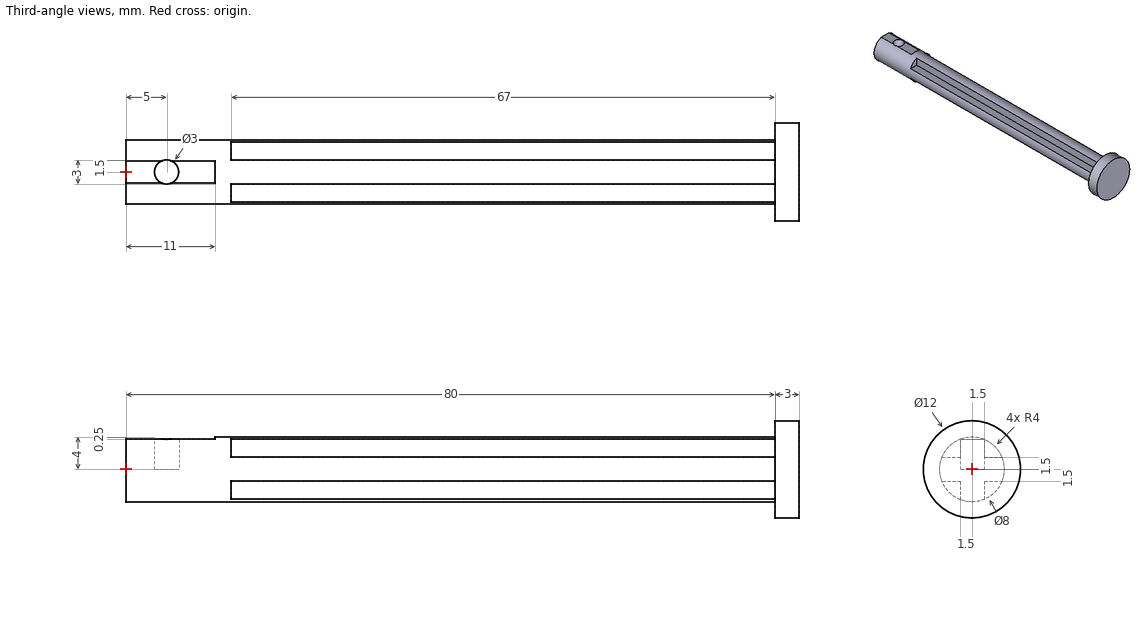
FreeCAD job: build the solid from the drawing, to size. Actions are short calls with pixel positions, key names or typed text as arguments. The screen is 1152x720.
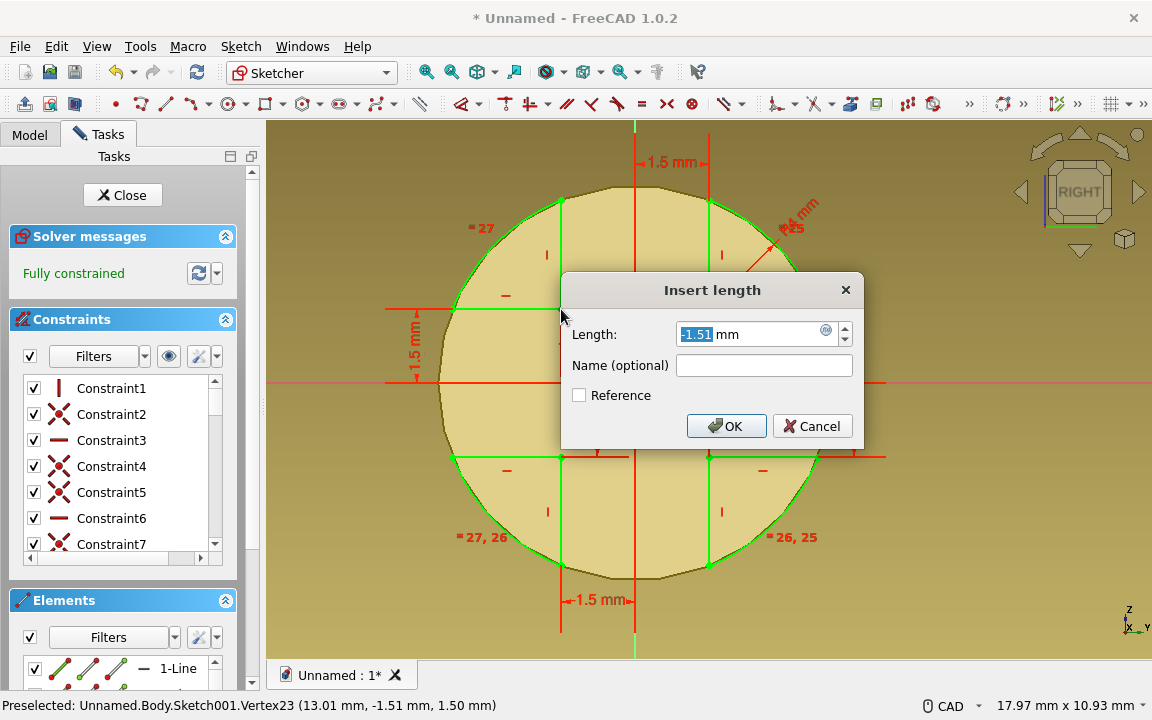
text(-1.5)
key(Return)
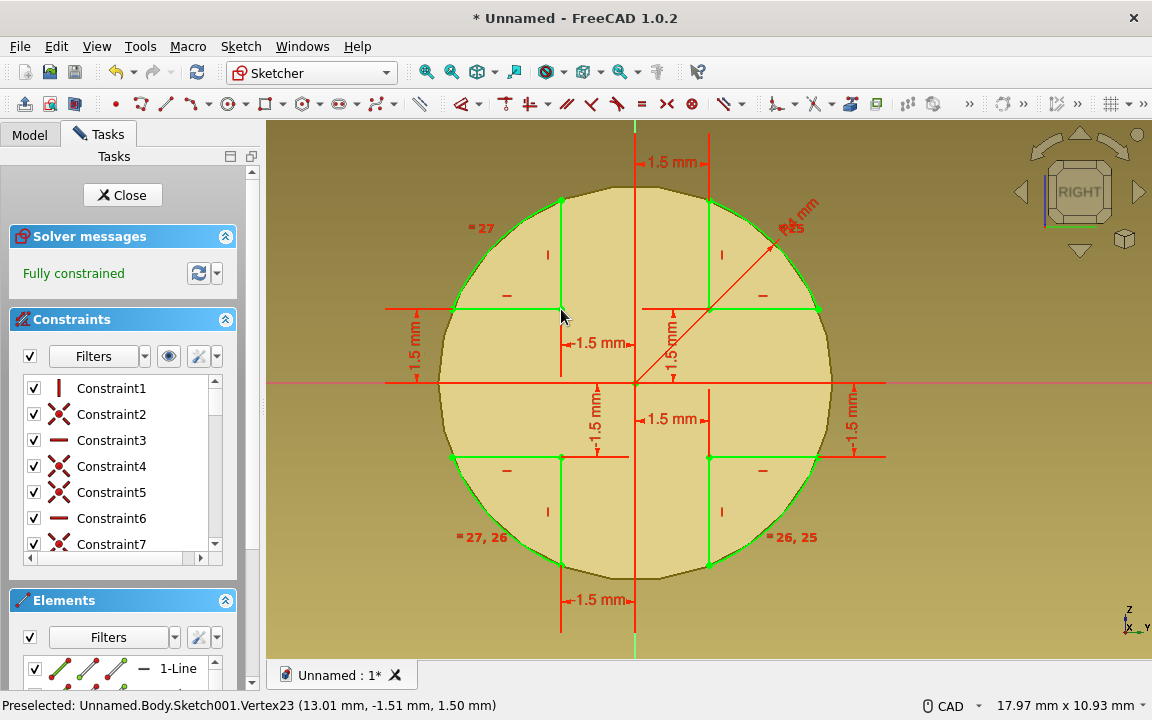
click(123, 195)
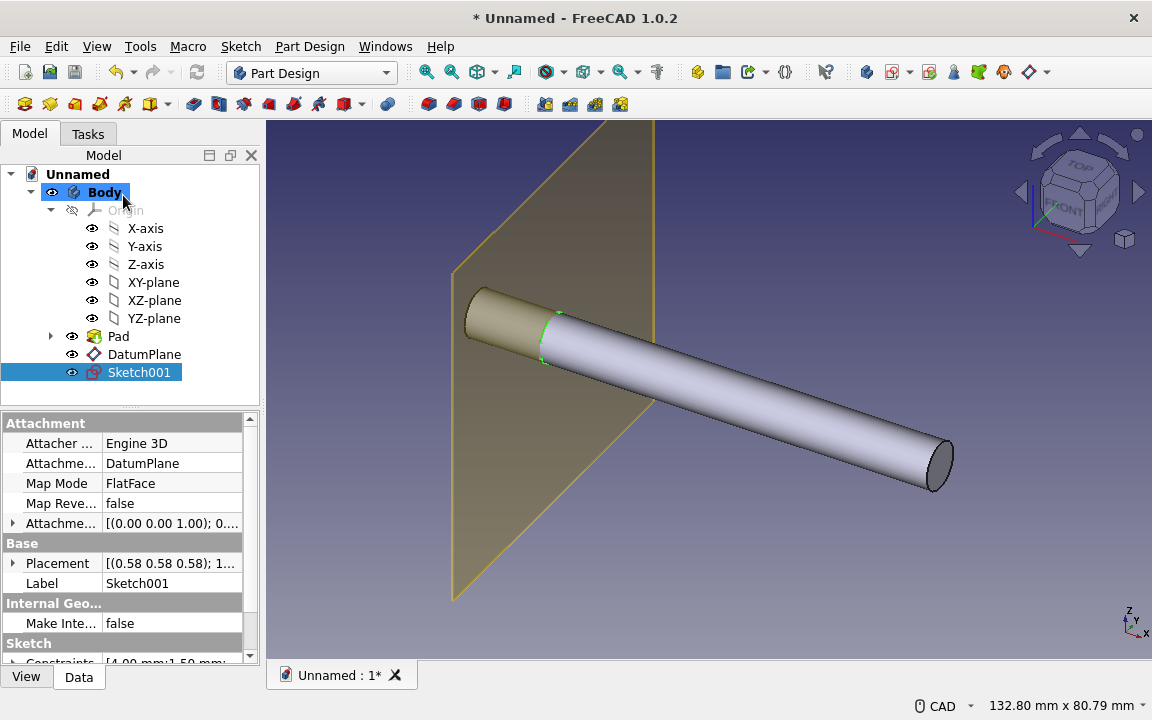
click(194, 104)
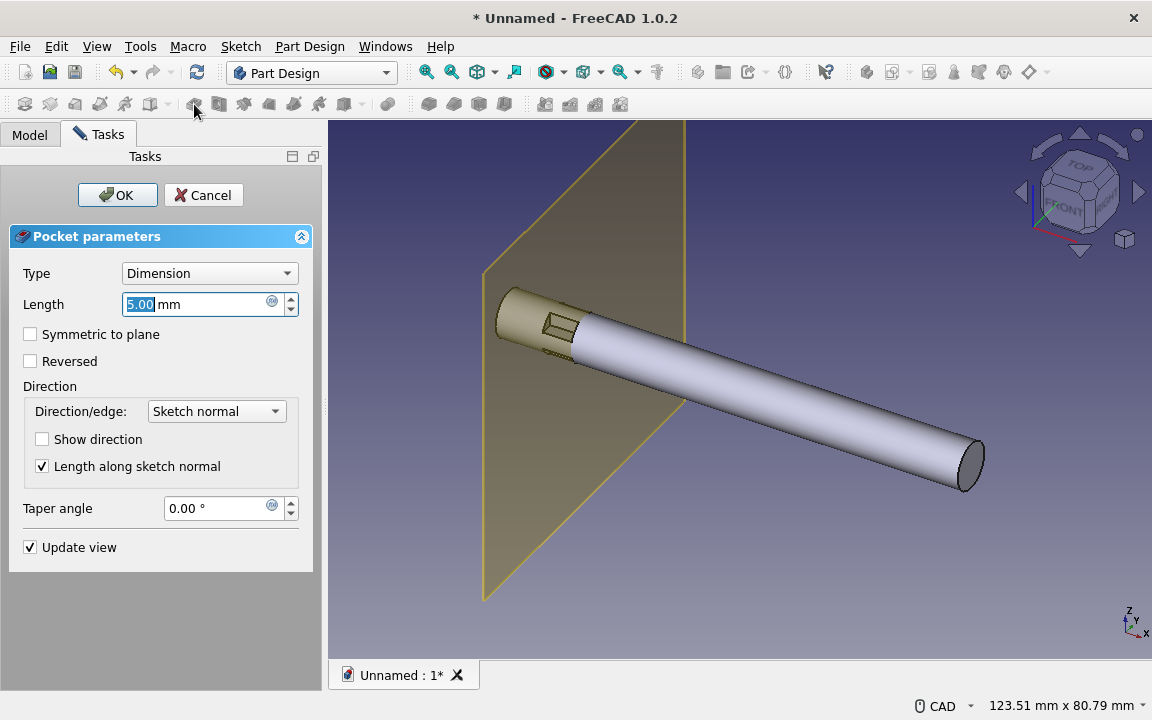
text(67)
key(Tab)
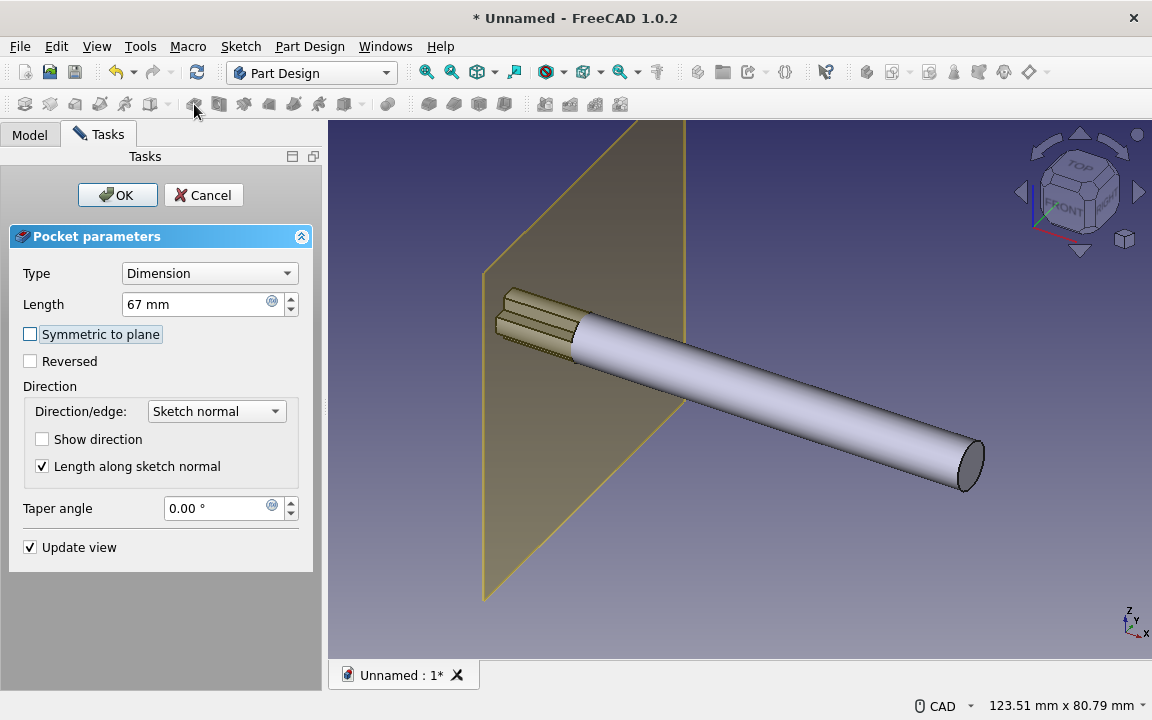
click(31, 361)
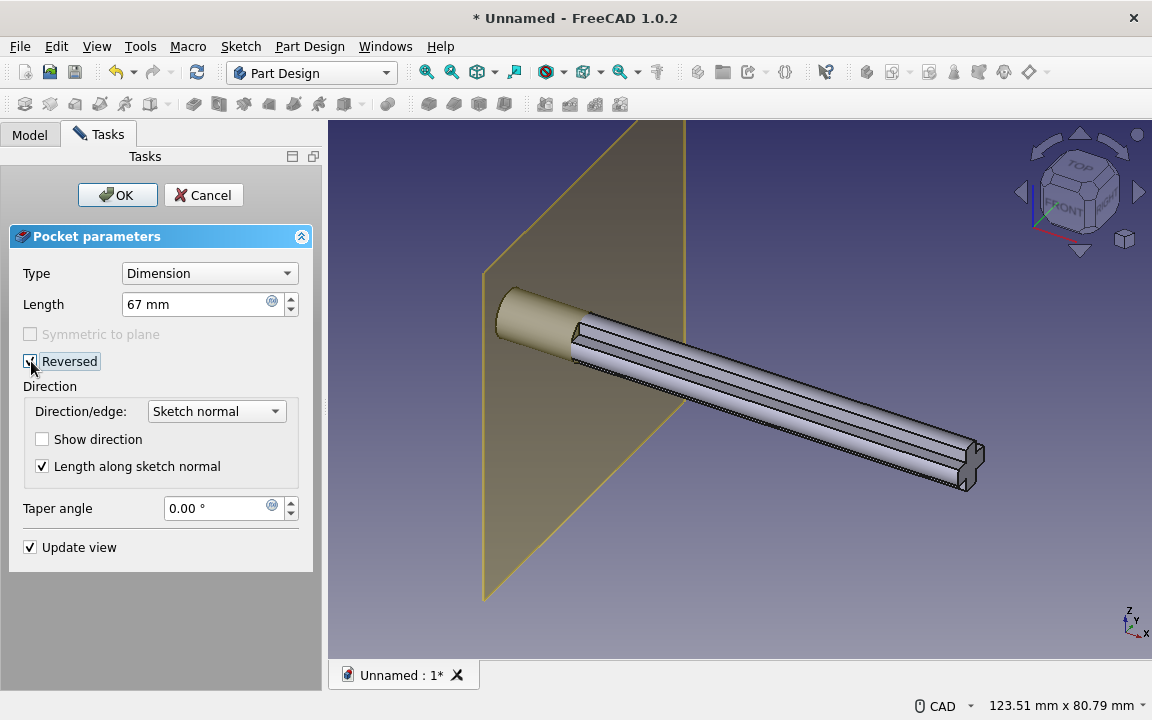
click(118, 195)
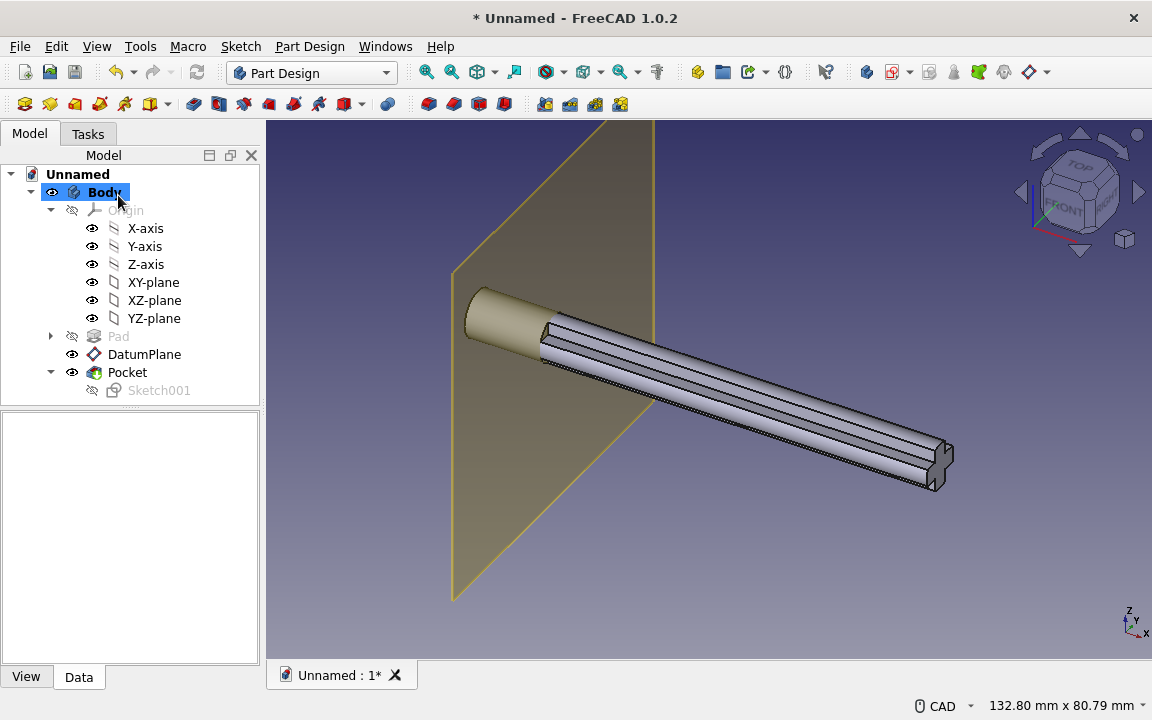
click(117, 354)
key(space)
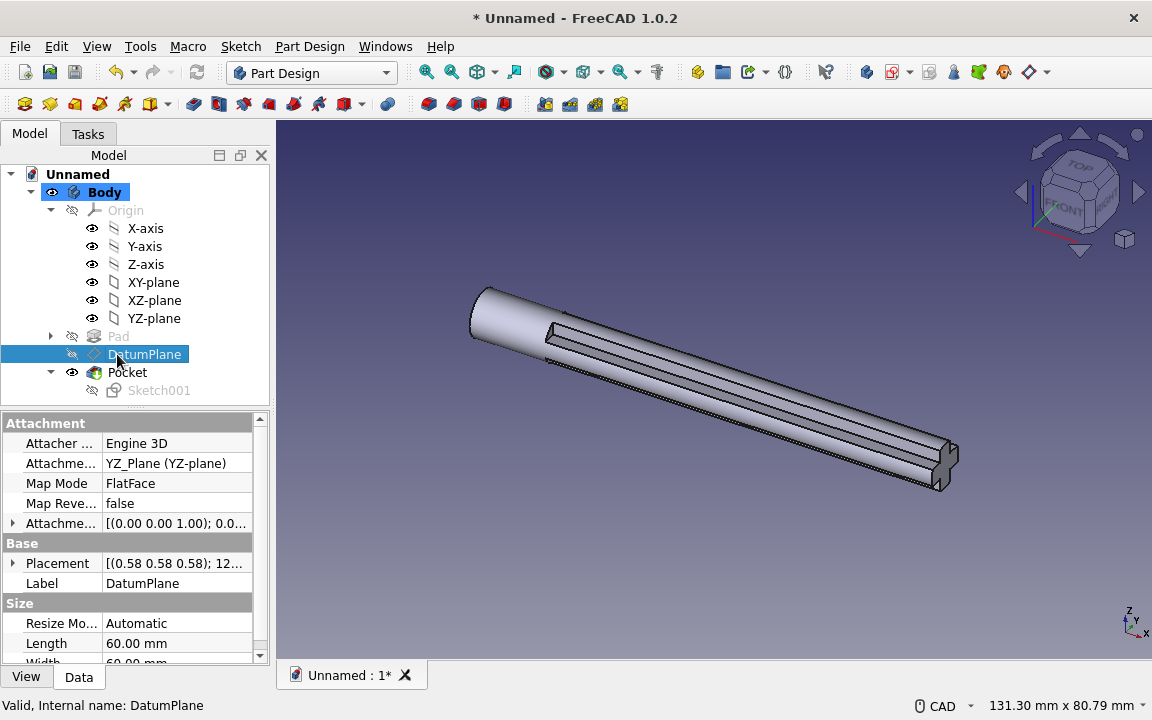
key(0)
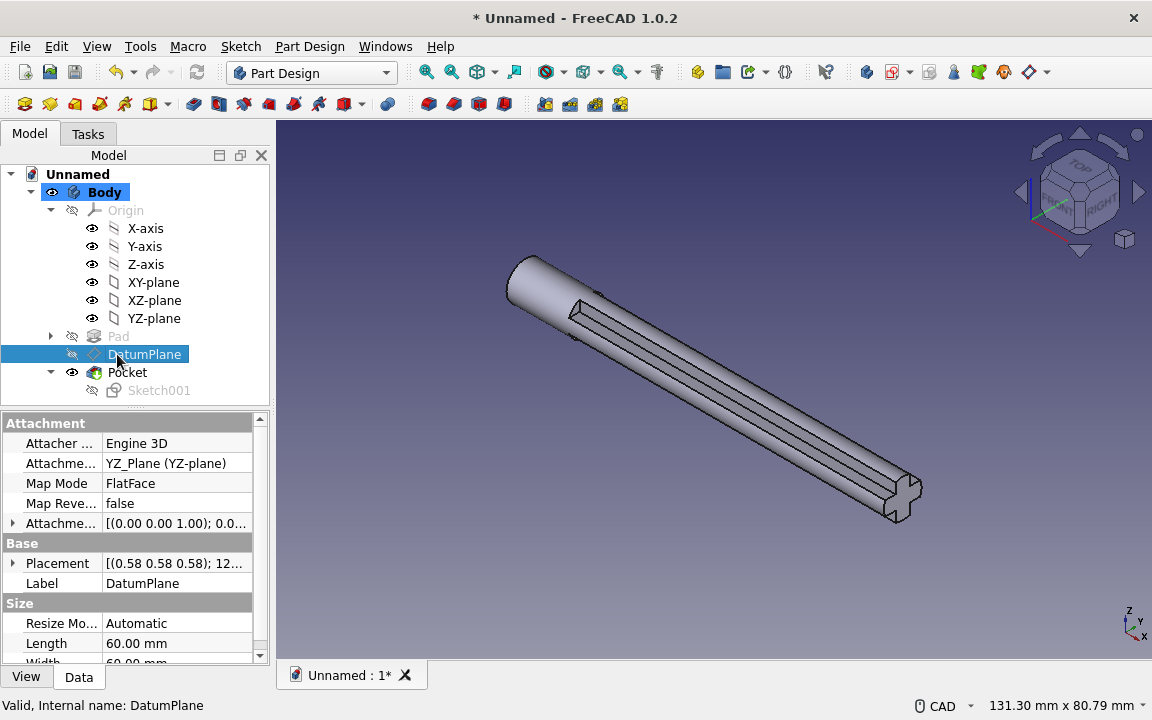
click(908, 494)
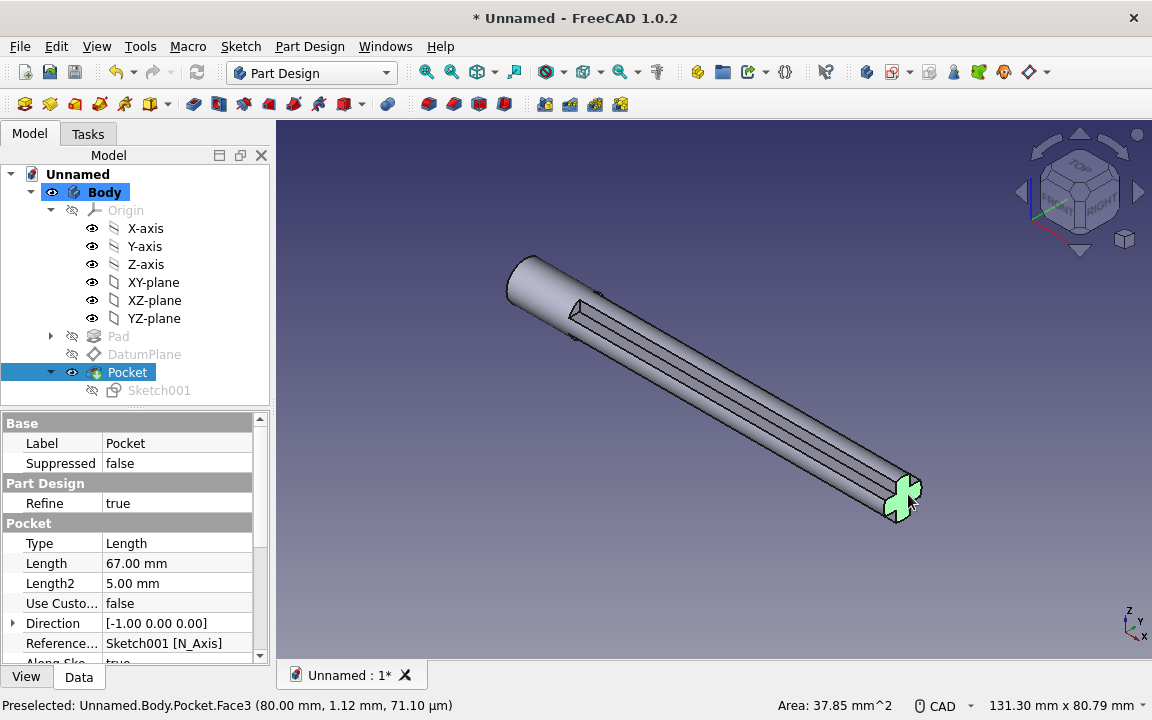
click(892, 72)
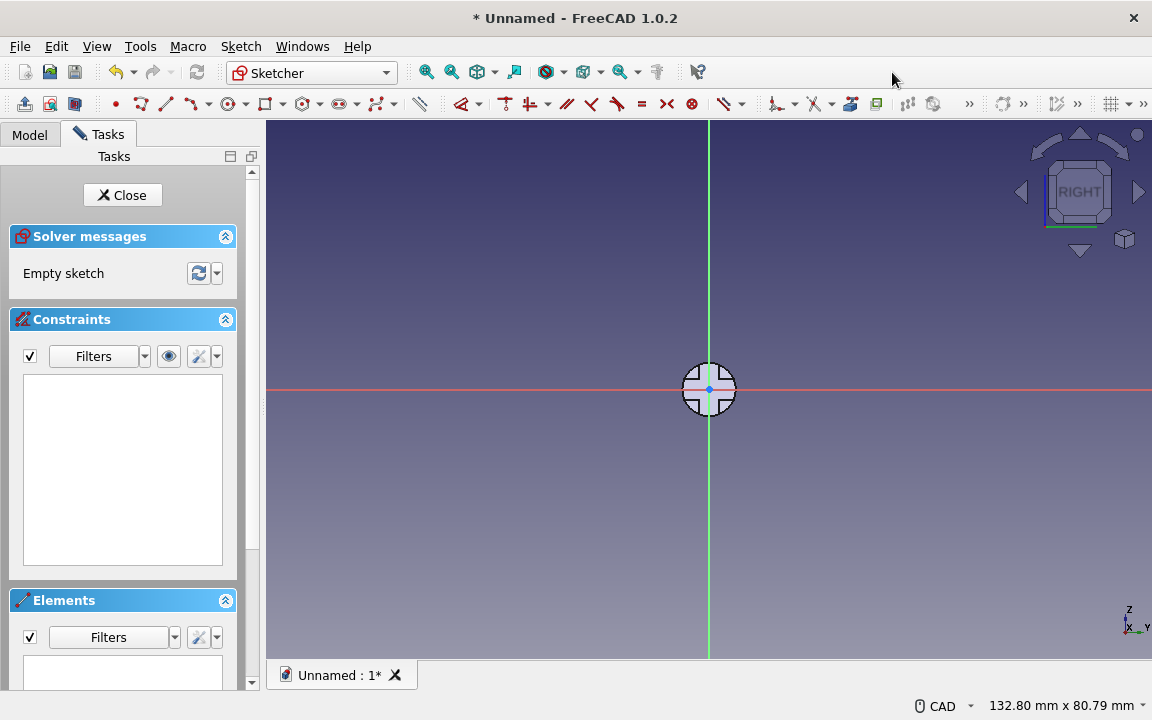
scroll(731, 389, up, 7)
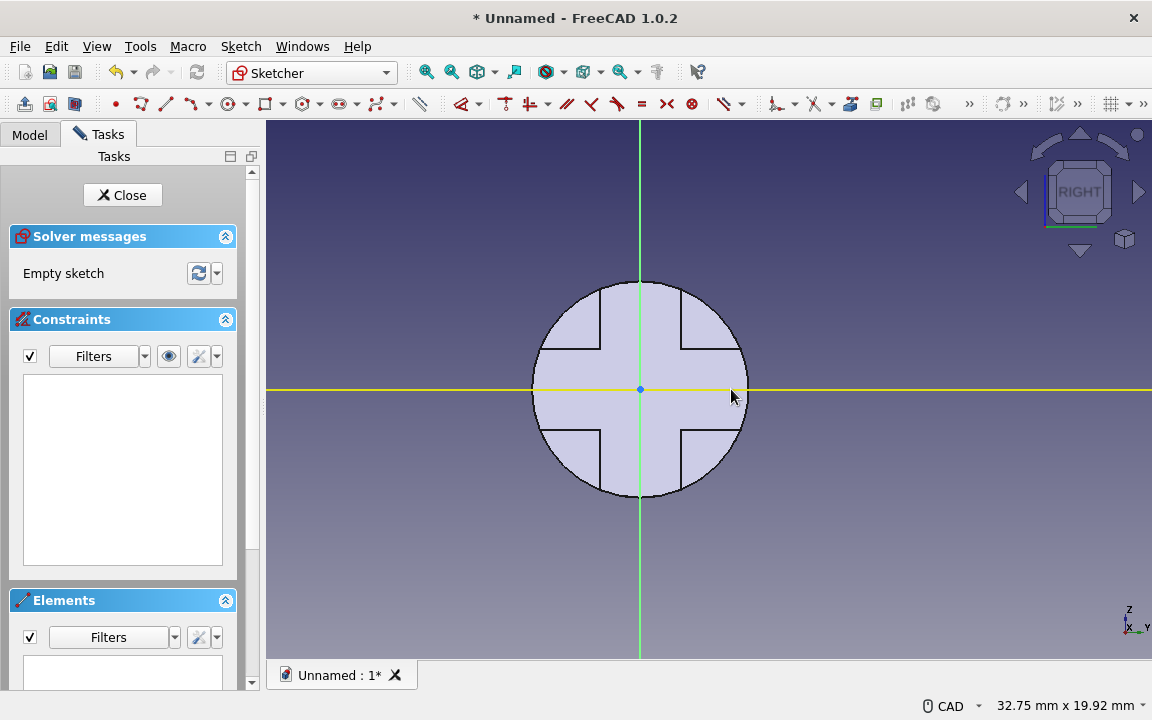
key(g)
key(c)